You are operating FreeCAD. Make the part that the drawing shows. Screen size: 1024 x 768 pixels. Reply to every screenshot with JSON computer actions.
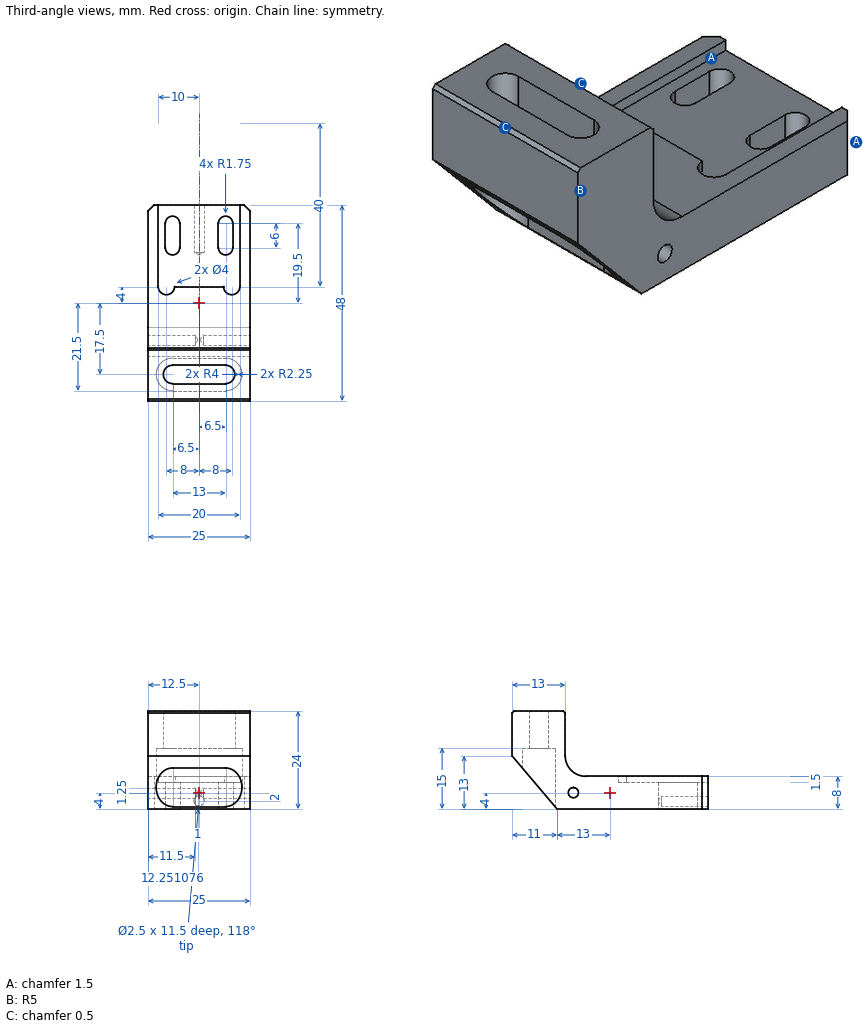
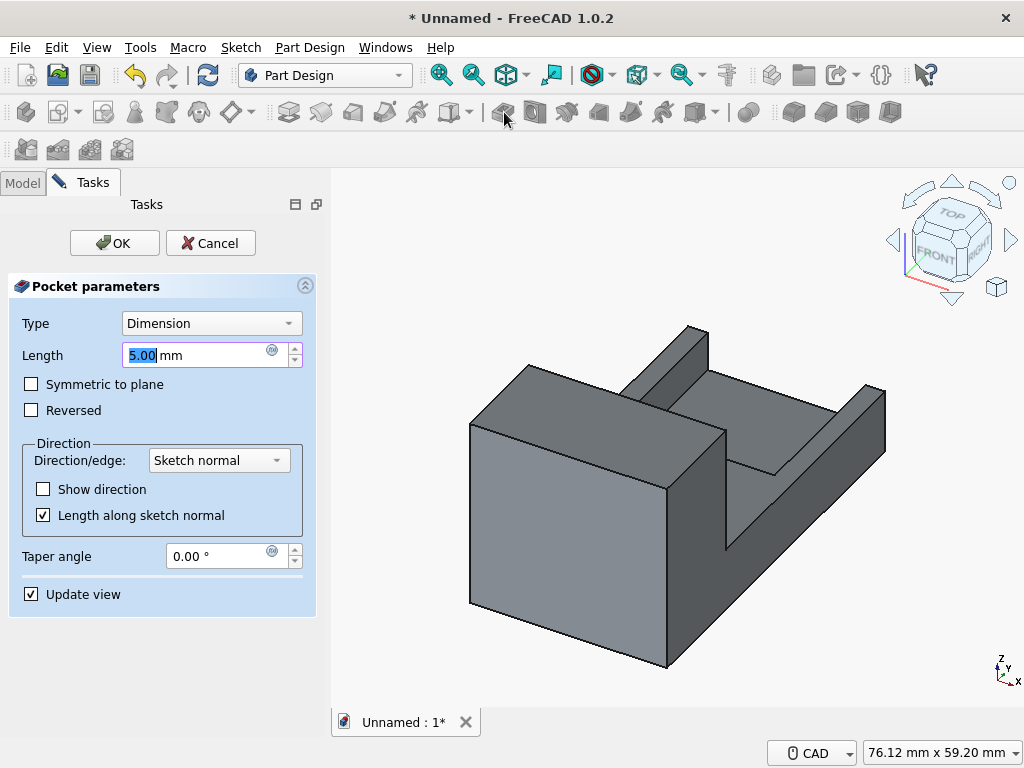
{"action": "type", "text": "1.5"}
{"action": "key", "text": "Tab"}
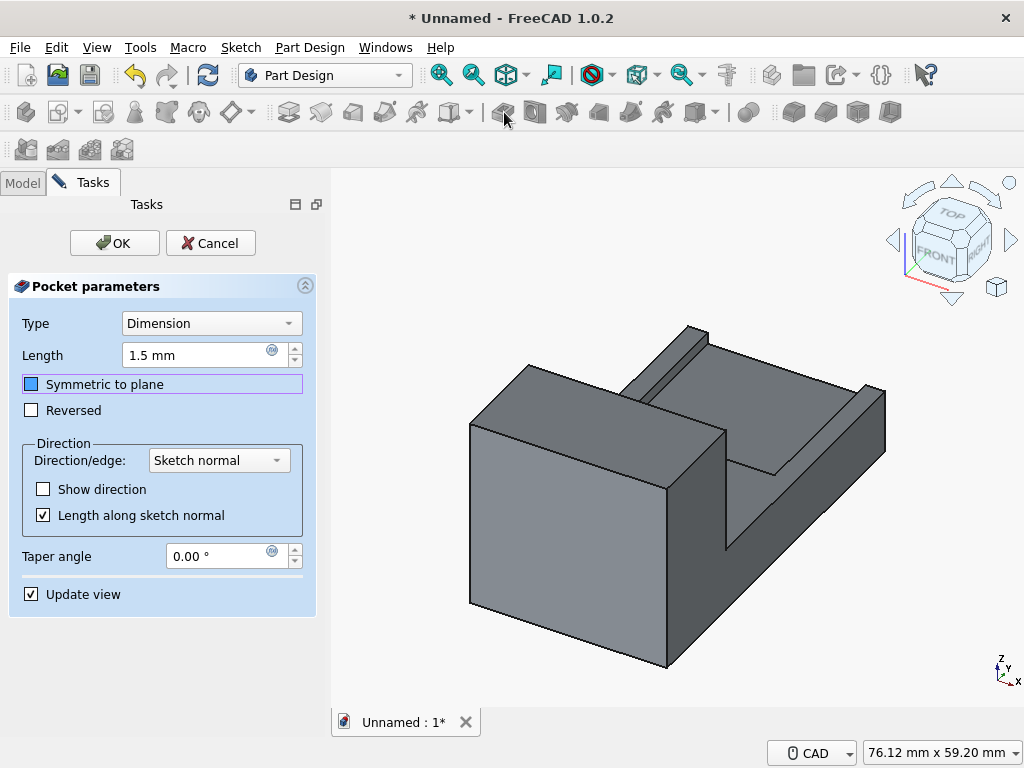
{"action": "left_click", "coordinate": [115, 243]}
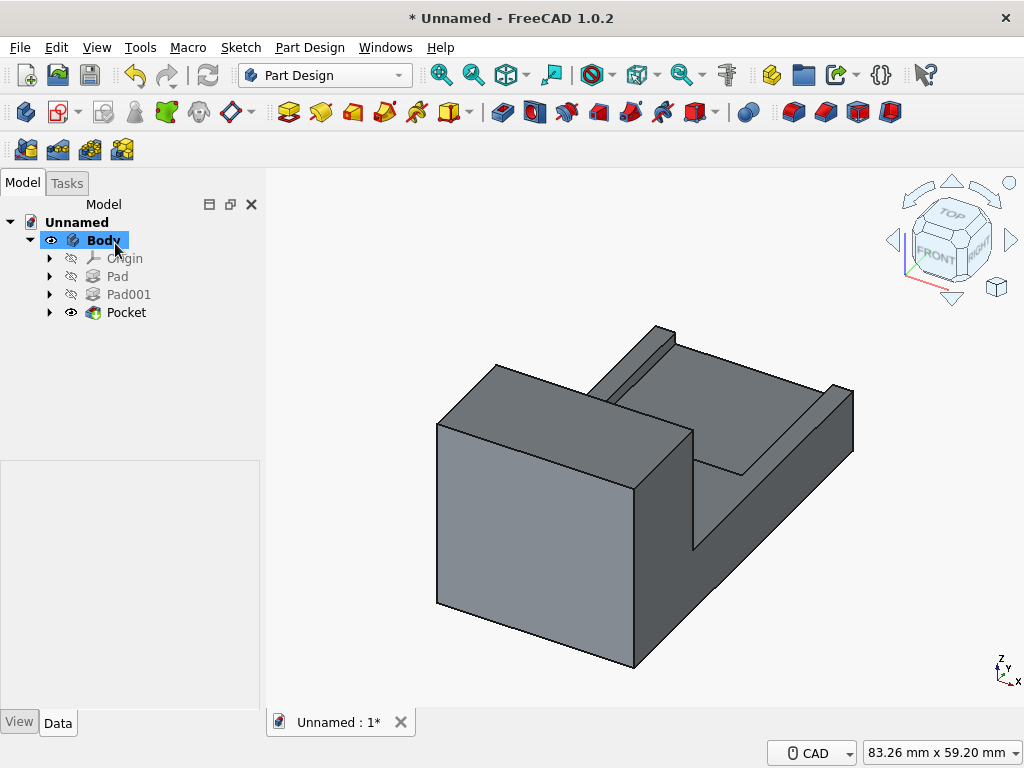
{"action": "key", "text": "4"}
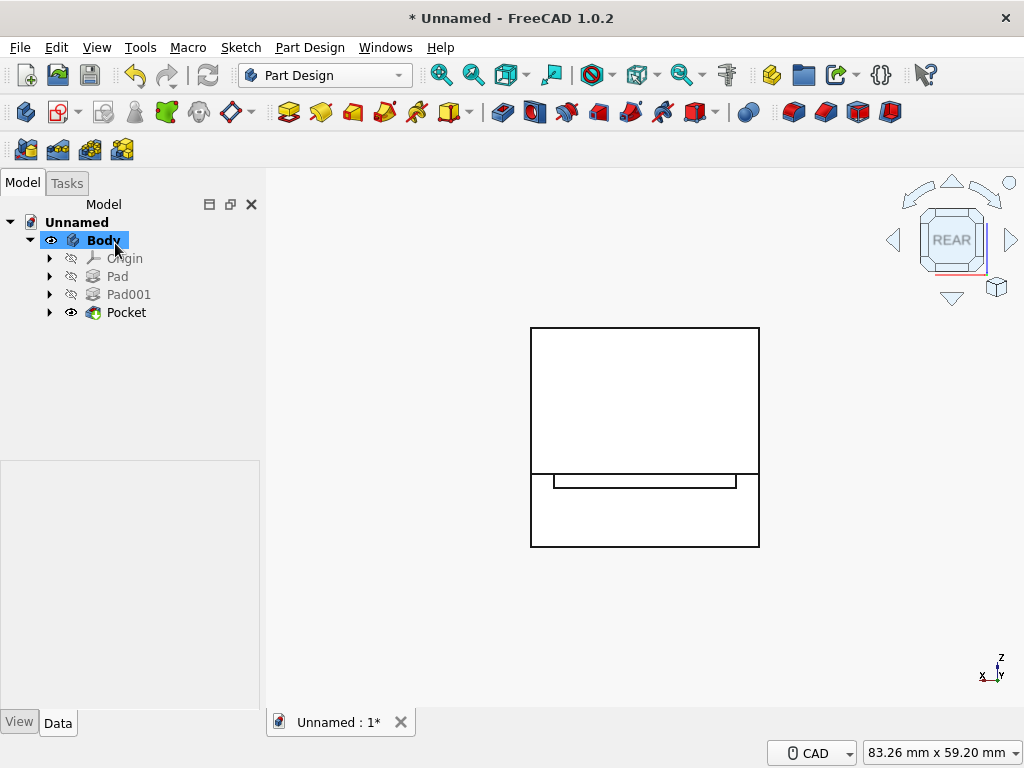
{"action": "left_click", "coordinate": [442, 76]}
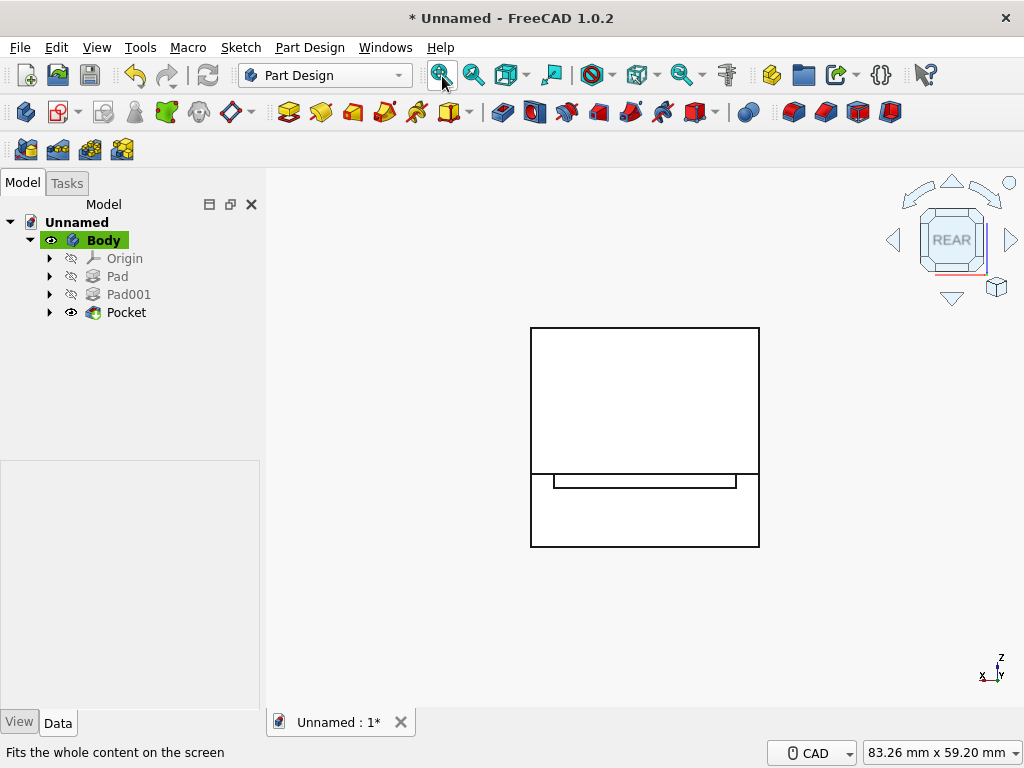
{"action": "left_click", "coordinate": [580, 520]}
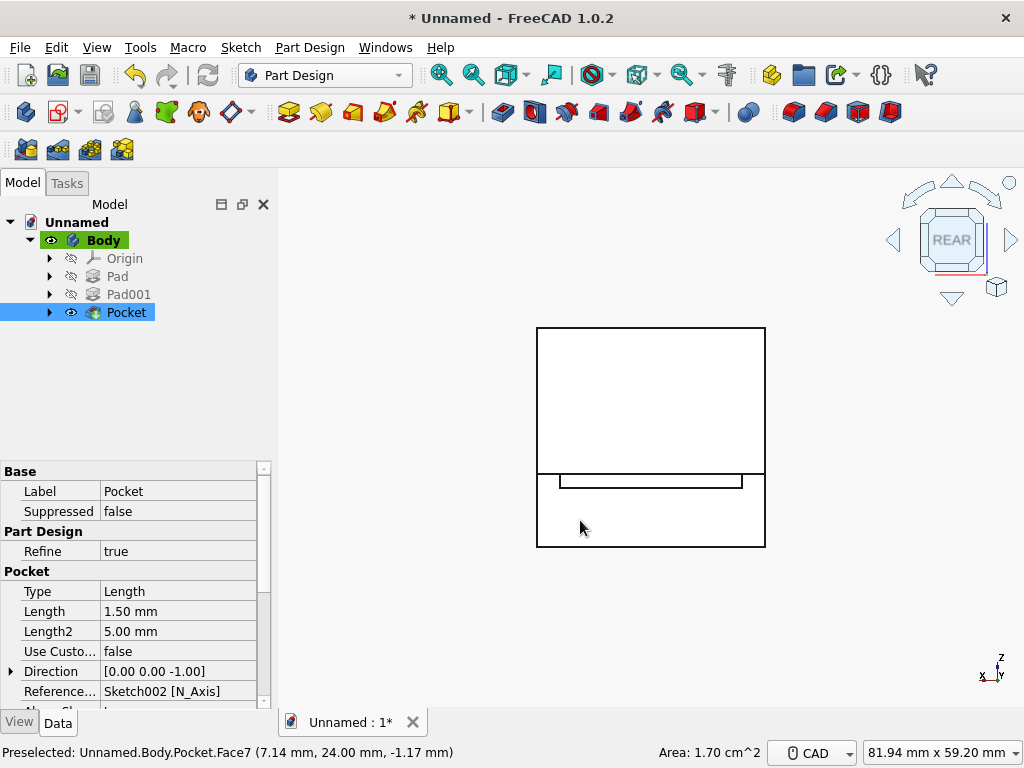
{"action": "left_click", "coordinate": [58, 112]}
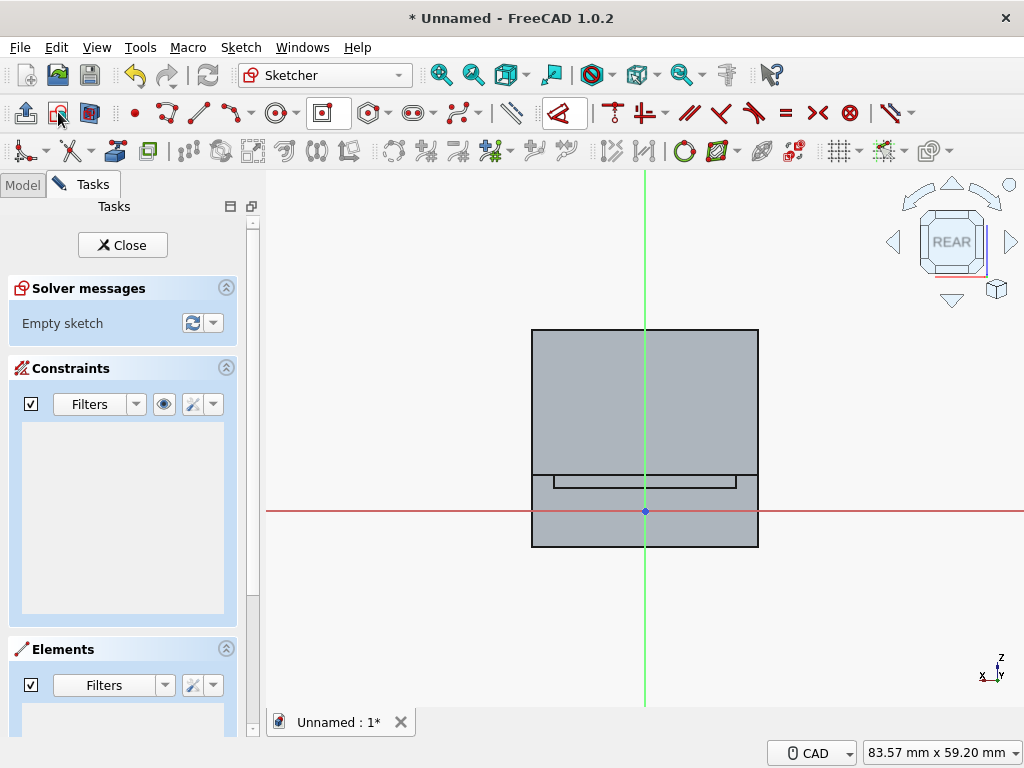
{"action": "scroll", "coordinate": [652, 535], "scroll_direction": "up", "scroll_amount": 12}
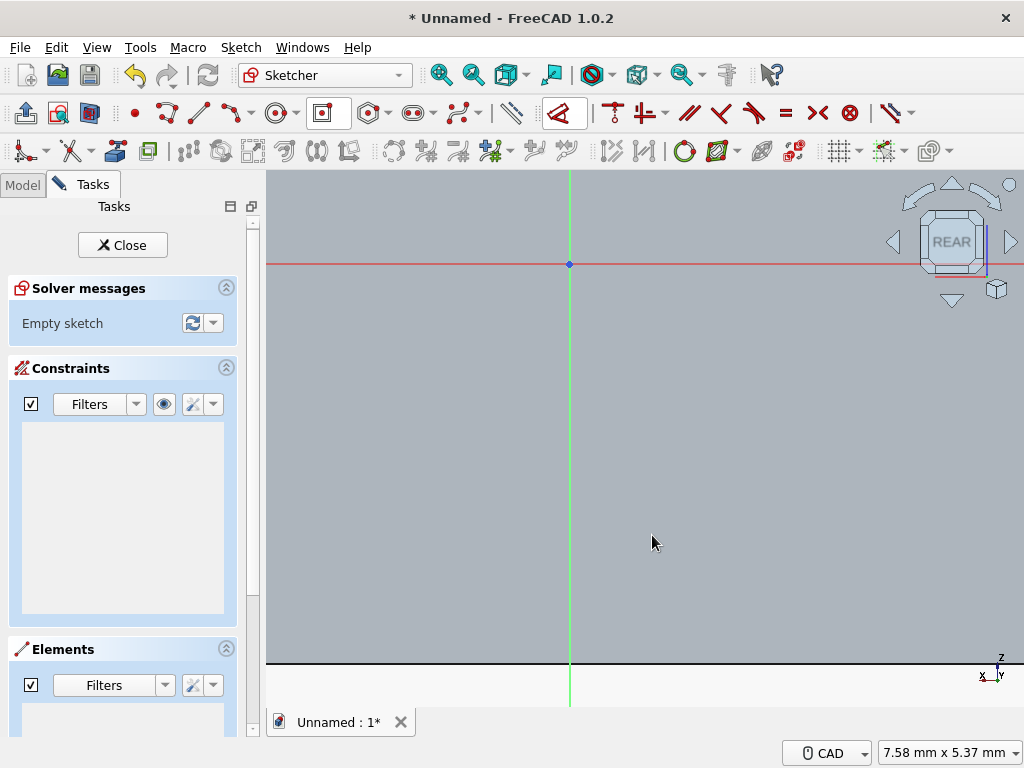
{"action": "left_click", "coordinate": [276, 114]}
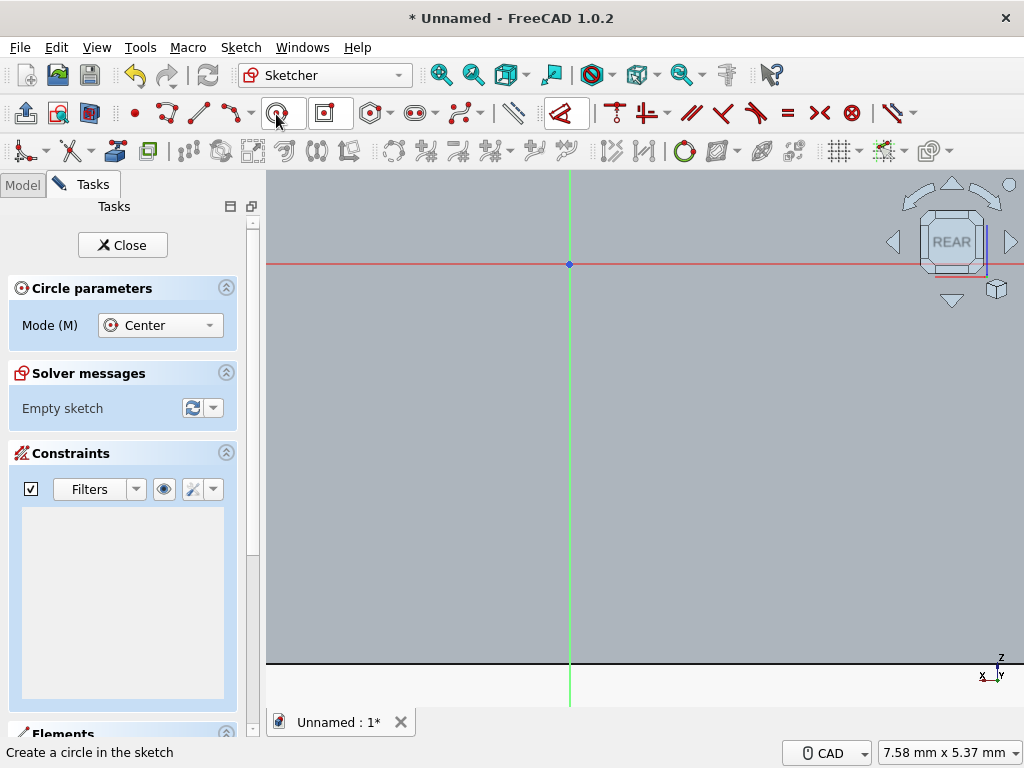
{"action": "left_click", "coordinate": [570, 464]}
{"action": "mouse_move", "coordinate": [658, 376]}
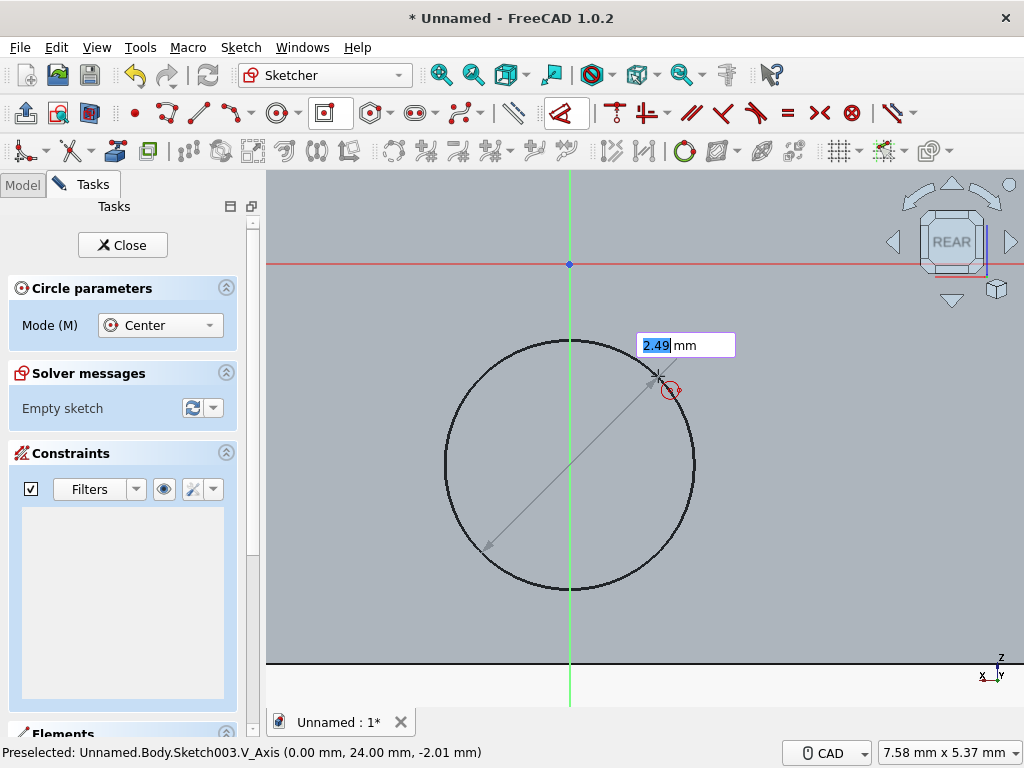
{"action": "type", "text": "2.5"}
{"action": "key", "text": "Return"}
{"action": "key", "text": "Escape"}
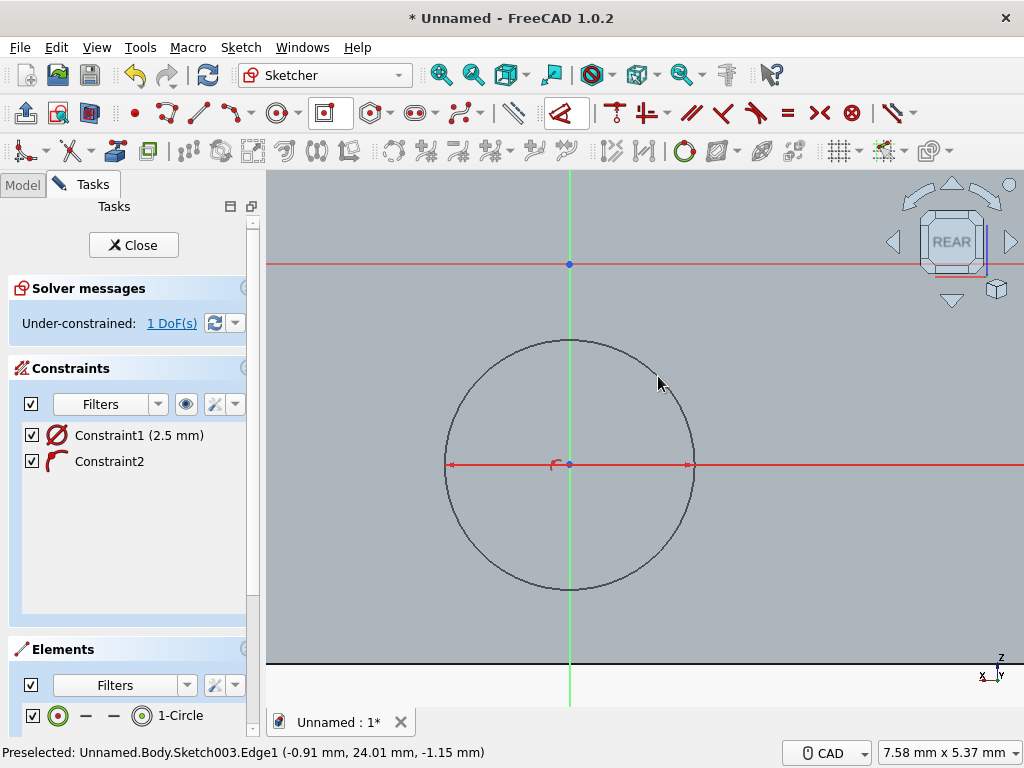
{"action": "left_click", "coordinate": [570, 465]}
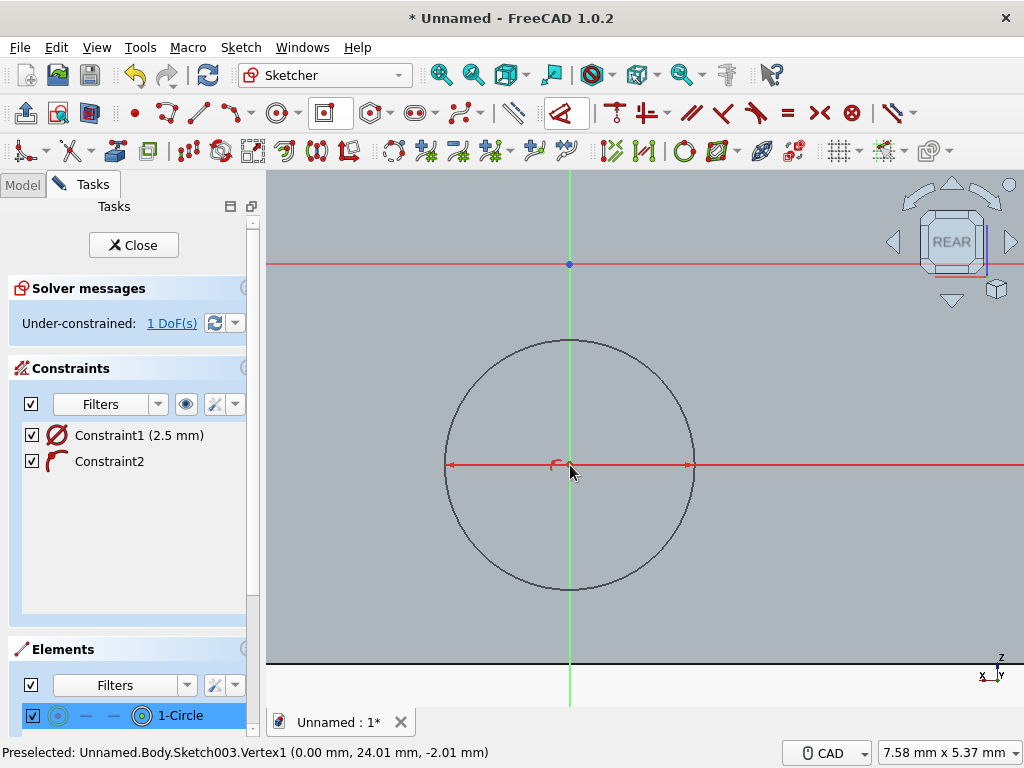
{"action": "left_click", "coordinate": [584, 114]}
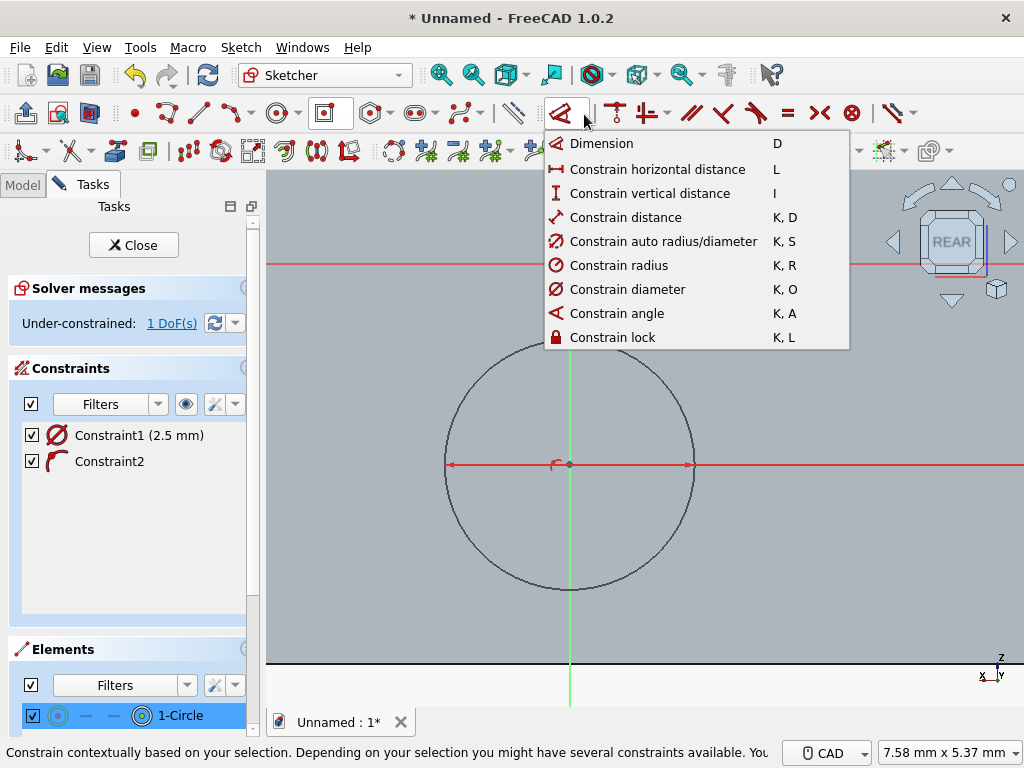
{"action": "left_click", "coordinate": [697, 193]}